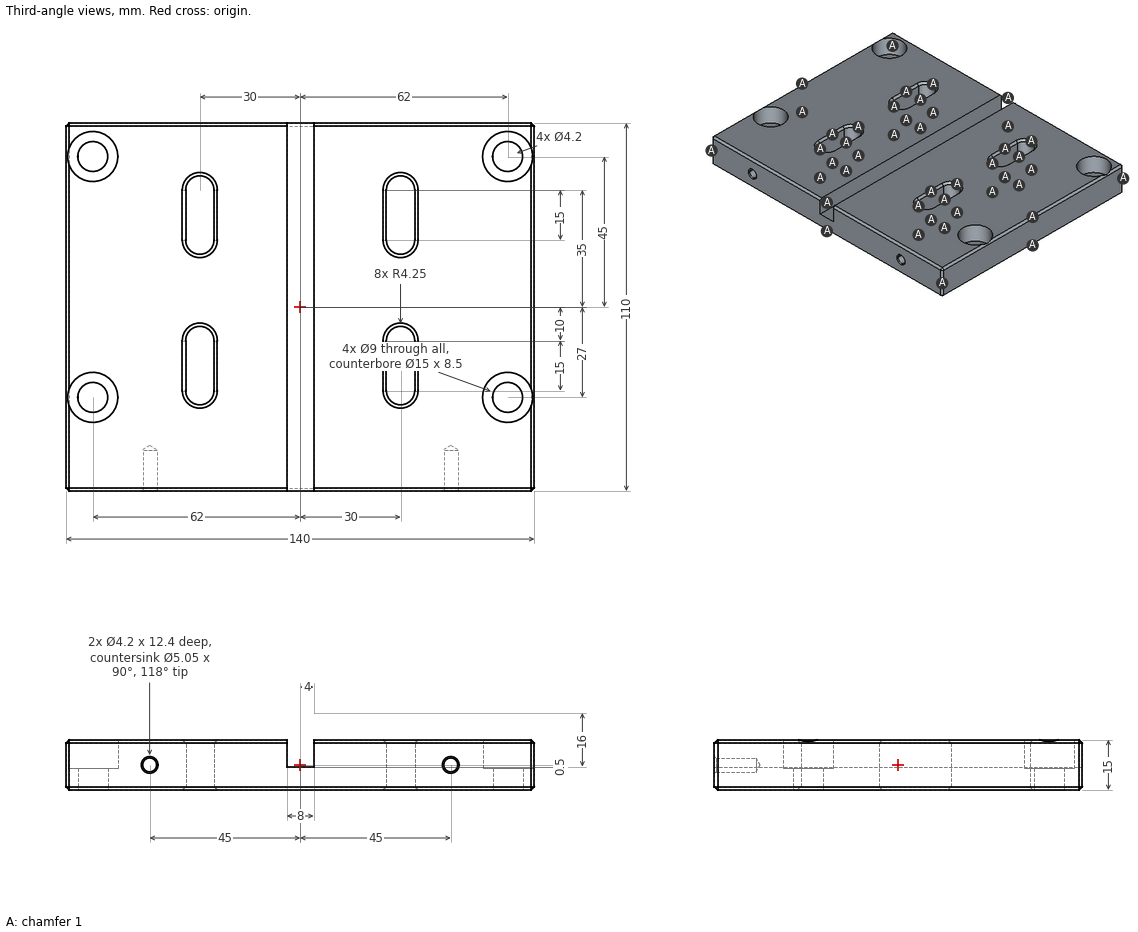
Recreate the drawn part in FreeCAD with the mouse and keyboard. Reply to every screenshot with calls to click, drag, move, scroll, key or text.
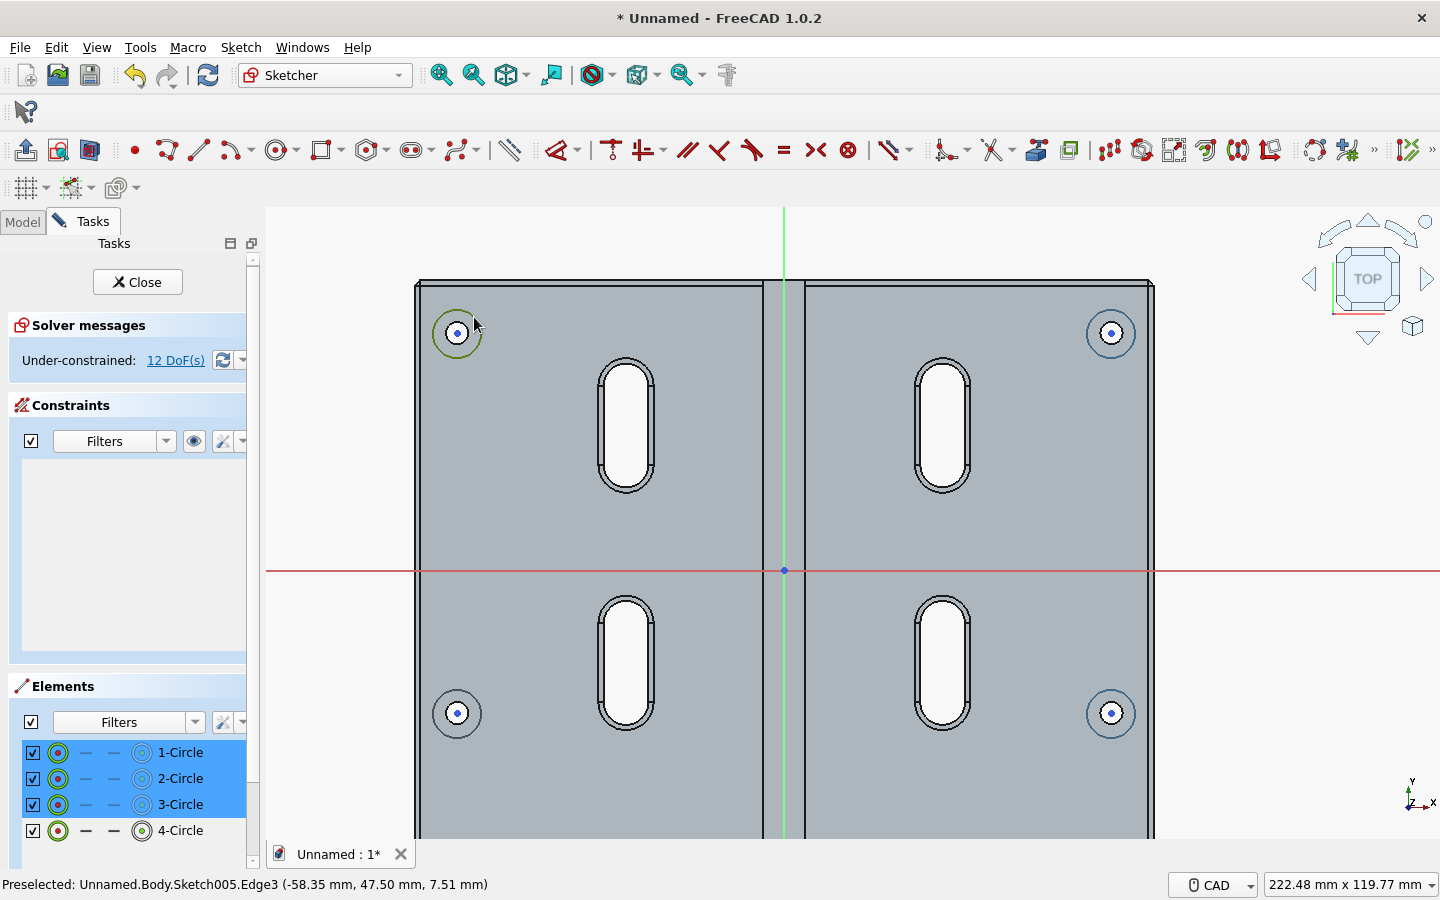
click(474, 697)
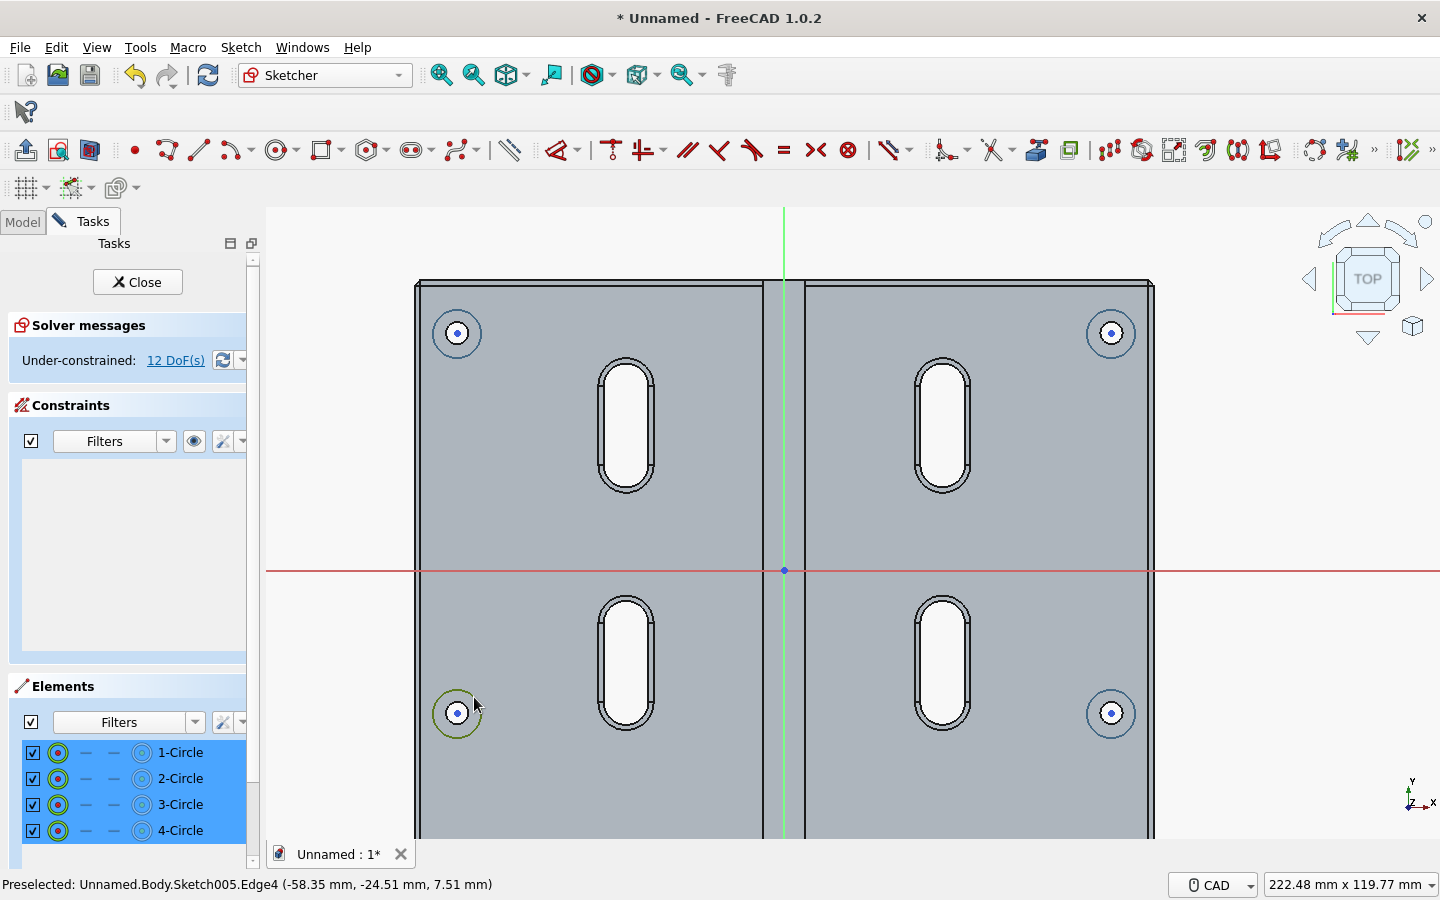
click(784, 150)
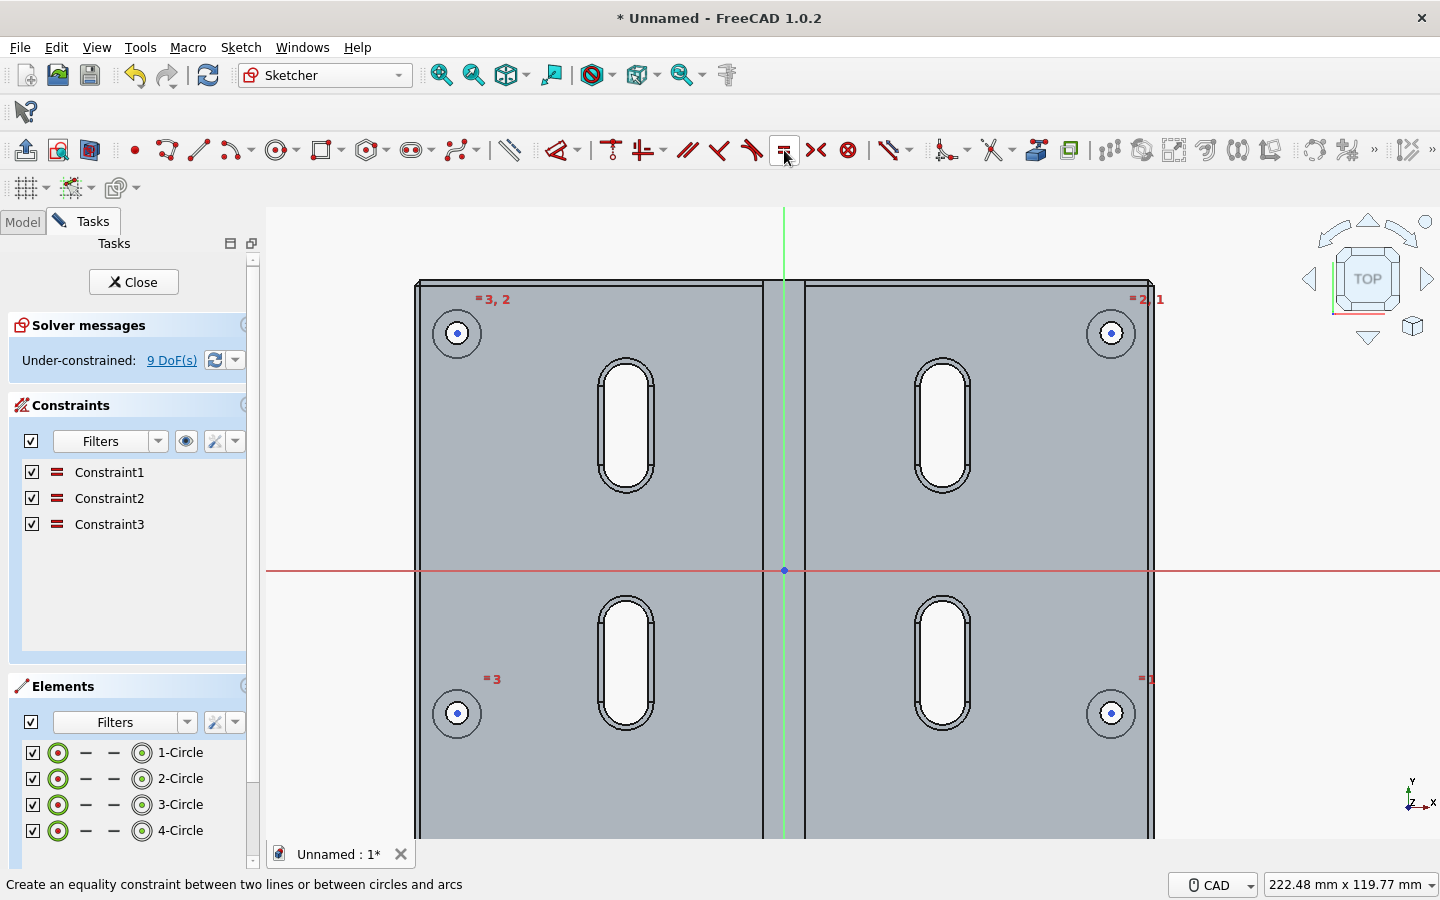
click(1111, 714)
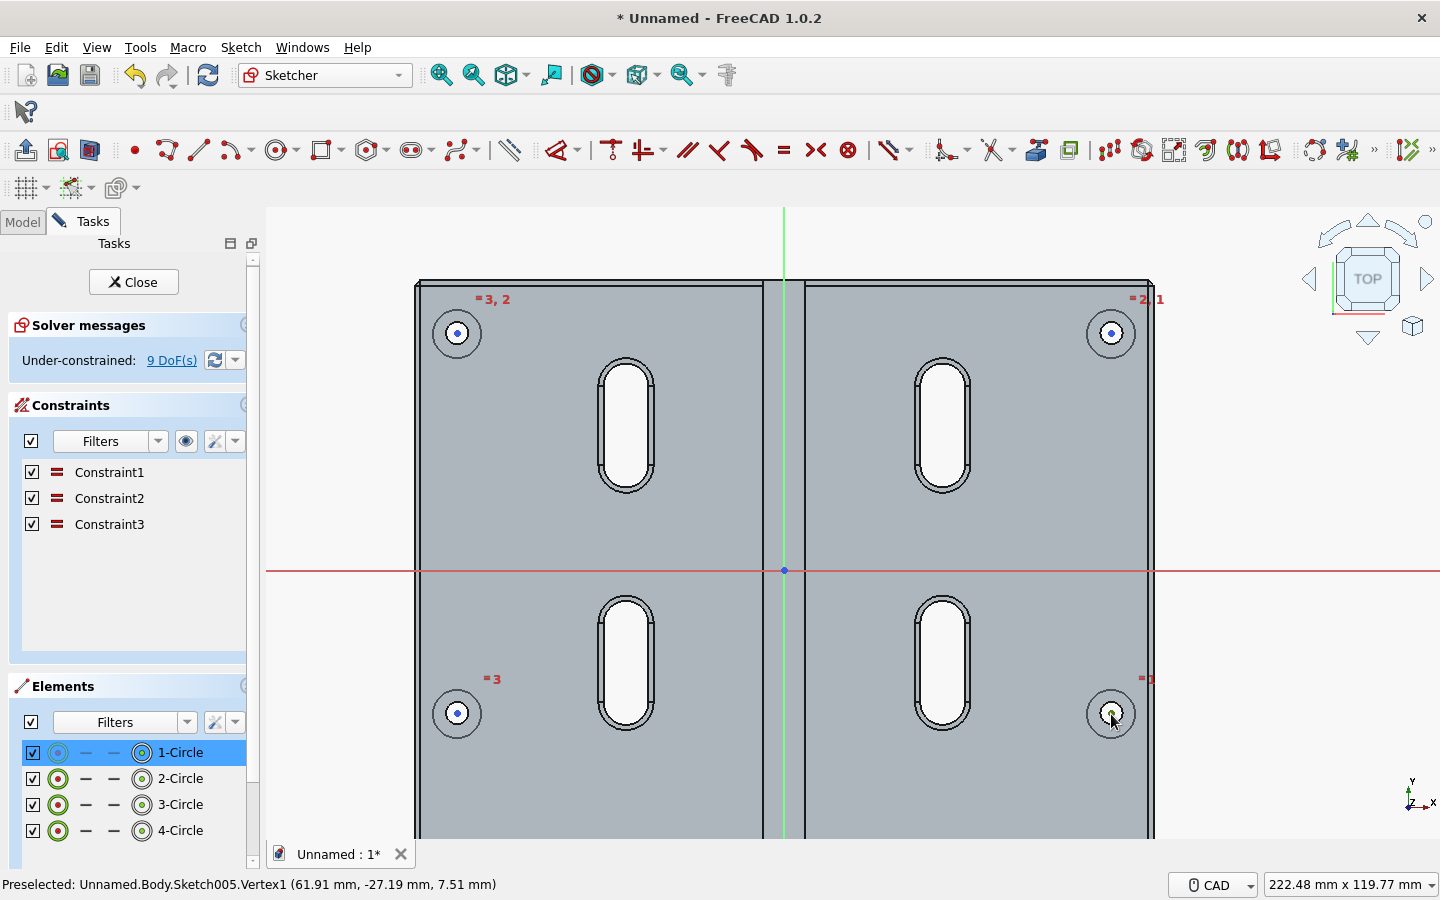
click(1111, 334)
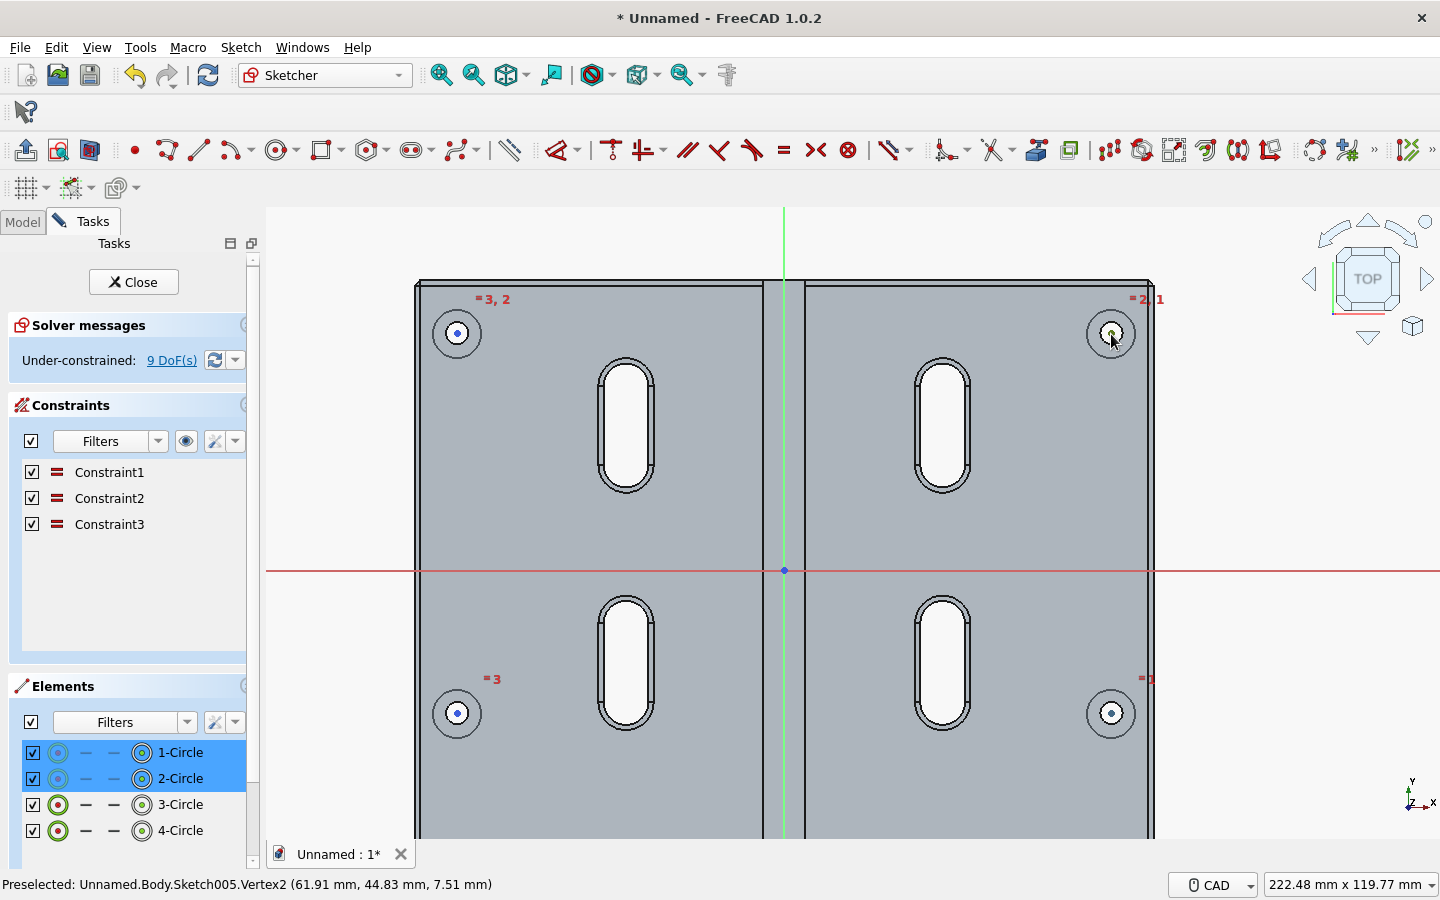
click(666, 150)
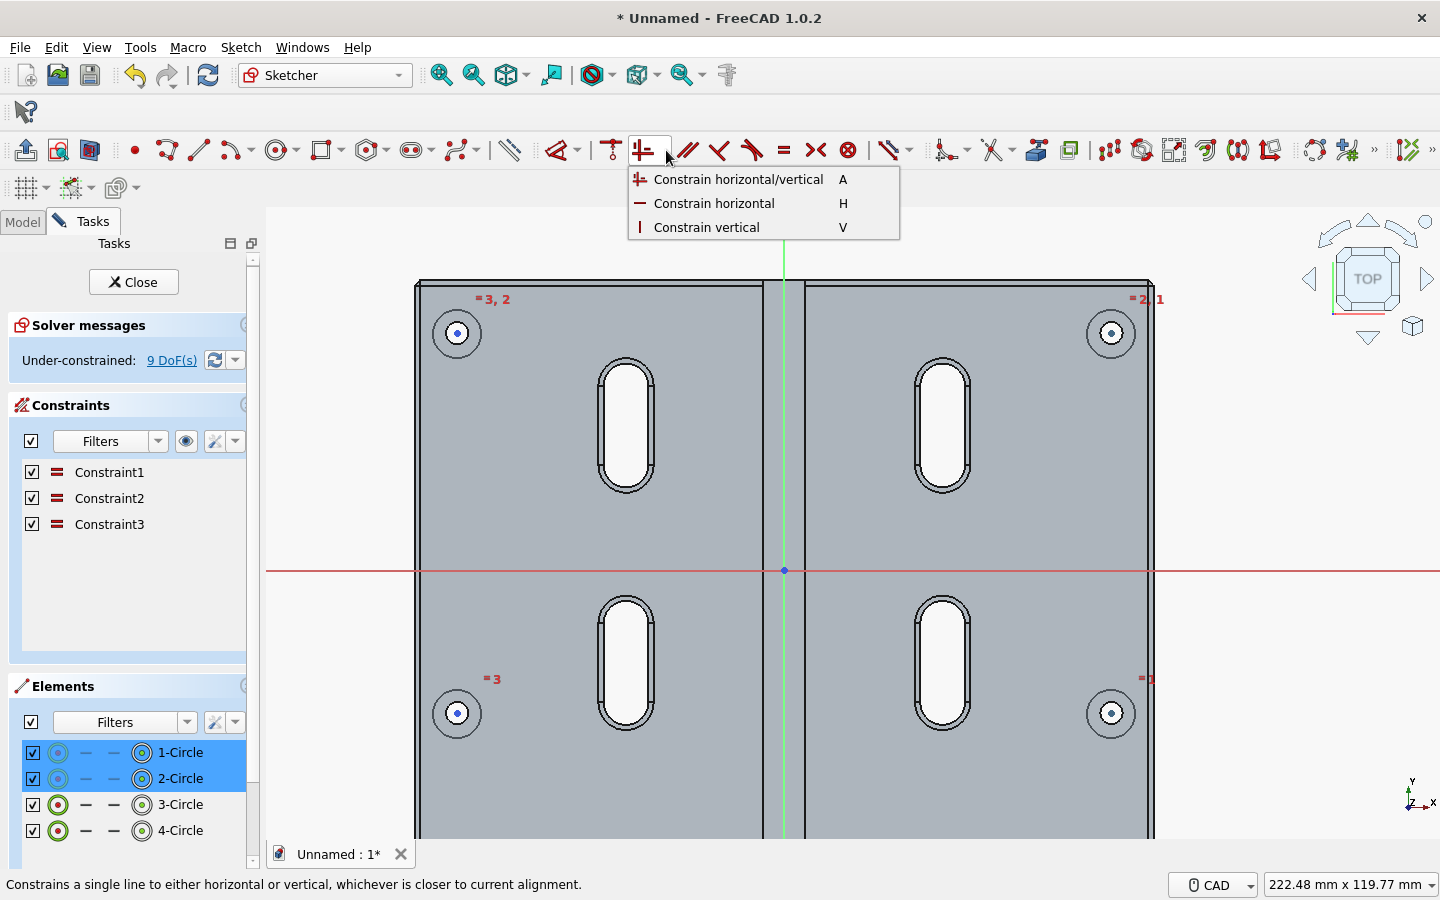
click(764, 227)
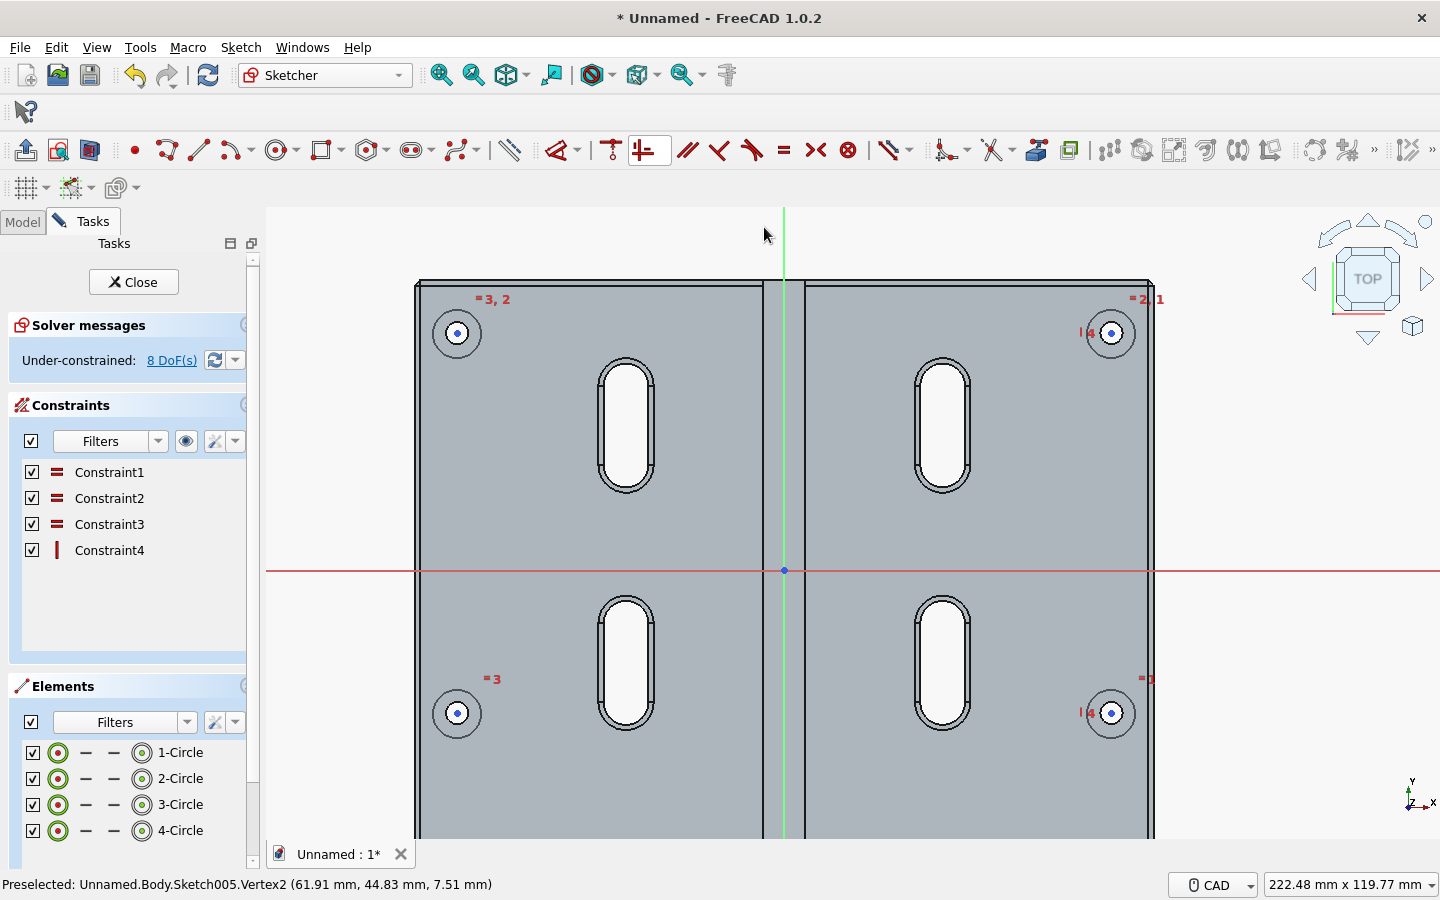
click(1111, 334)